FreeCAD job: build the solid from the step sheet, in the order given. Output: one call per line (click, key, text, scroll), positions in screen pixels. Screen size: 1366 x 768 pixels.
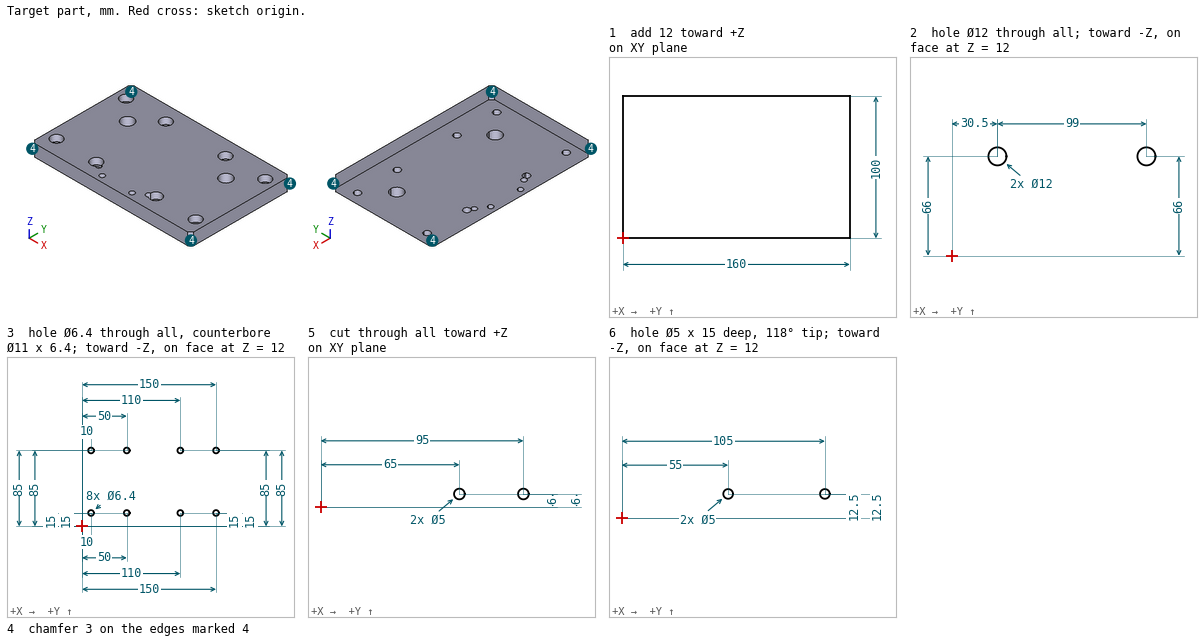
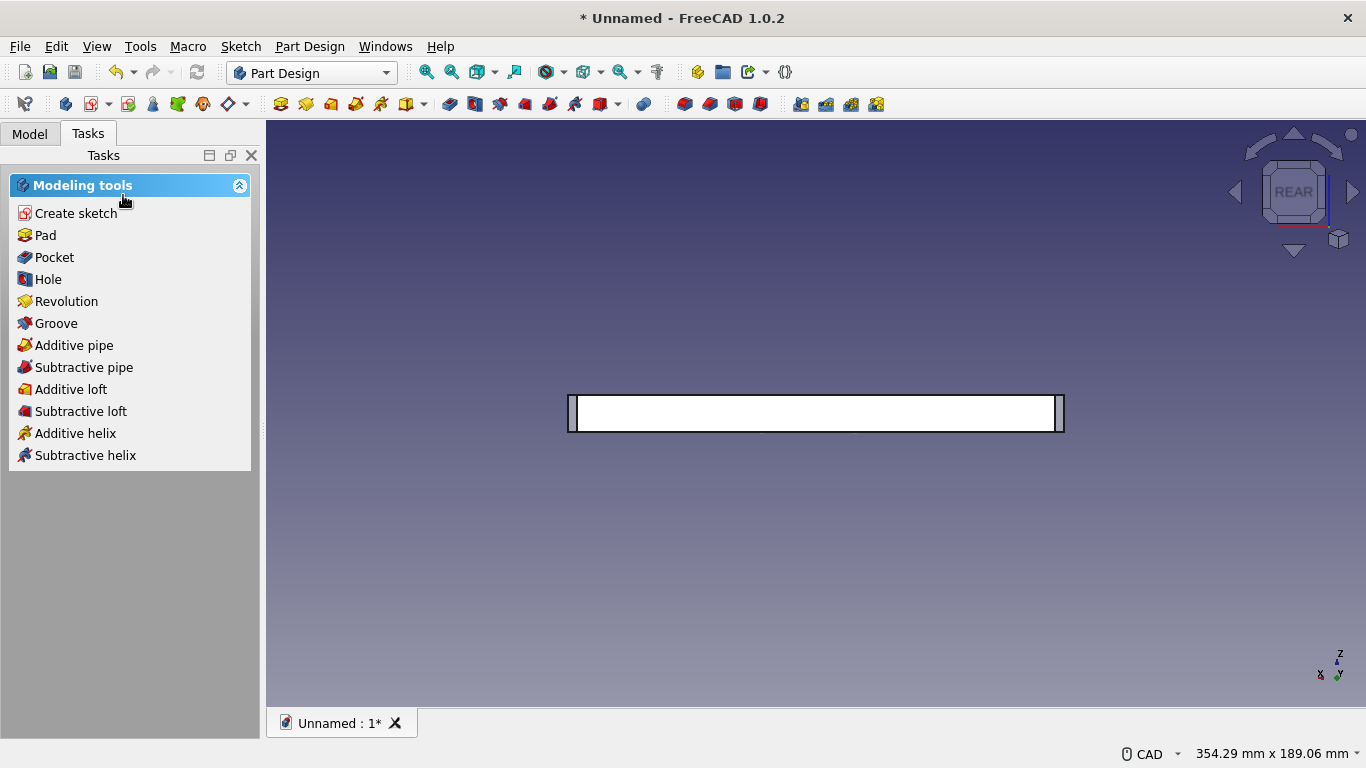
click(450, 104)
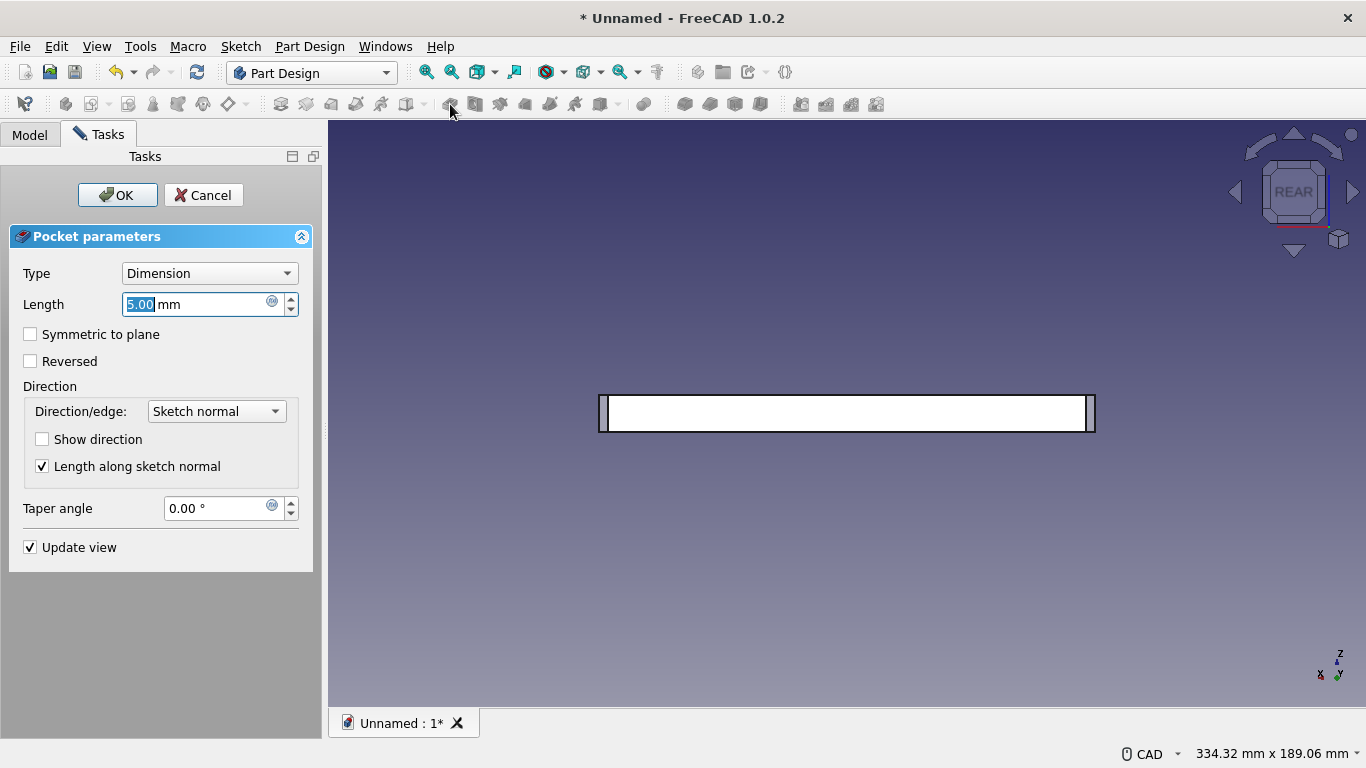
click(210, 274)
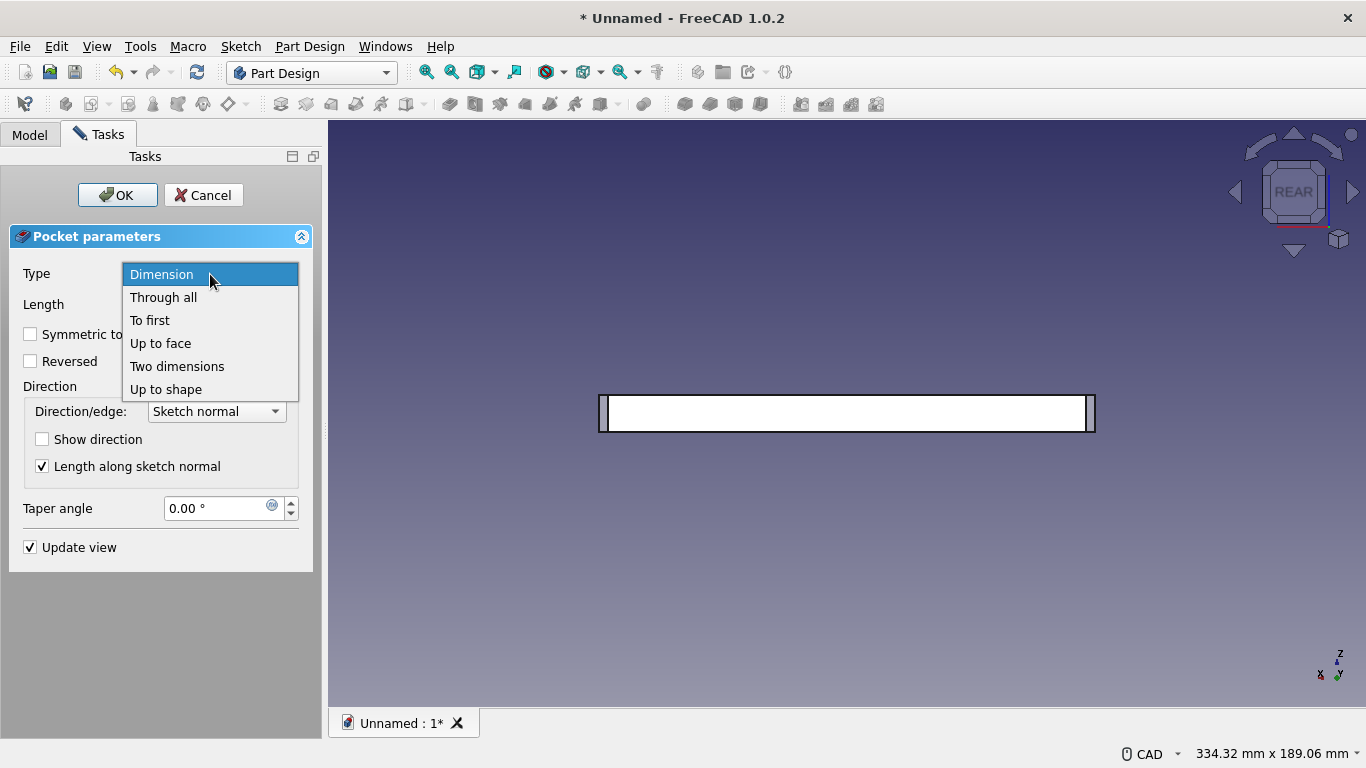
click(208, 298)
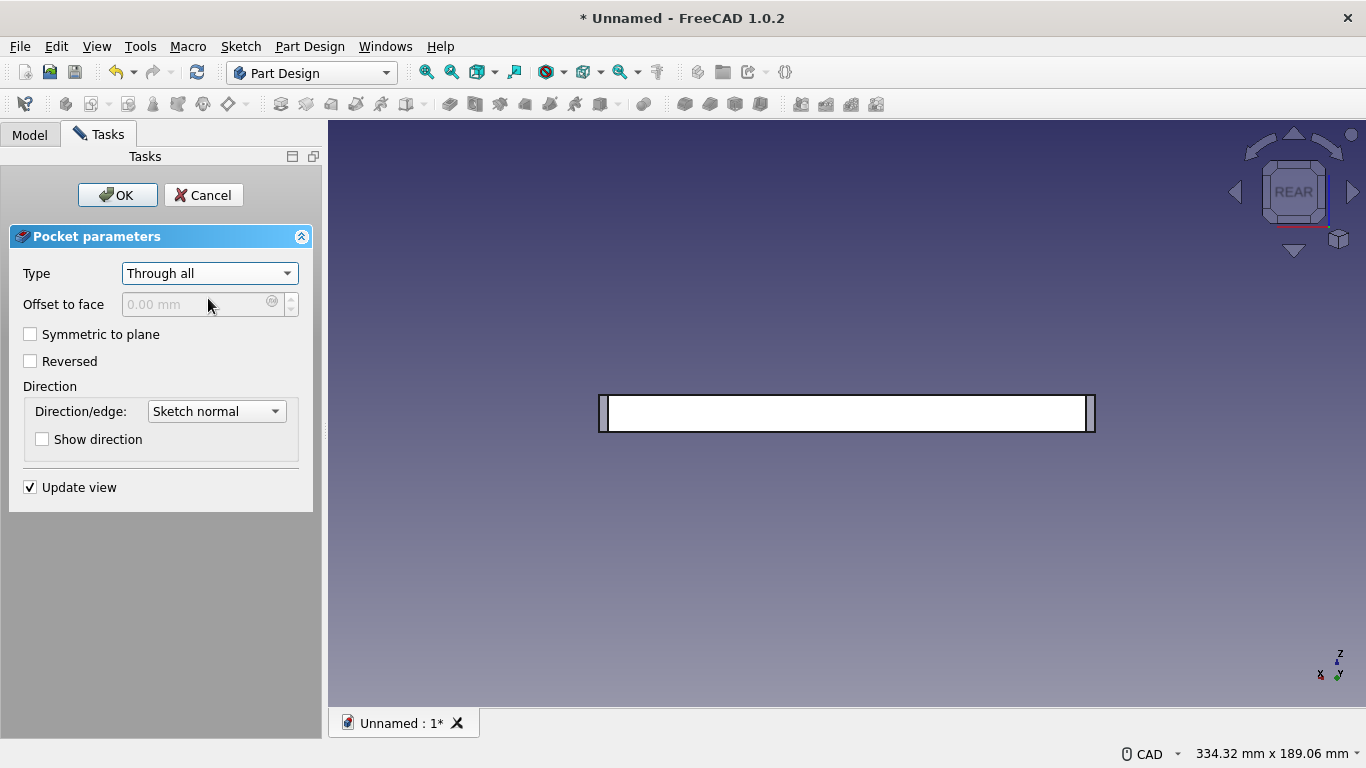
click(31, 361)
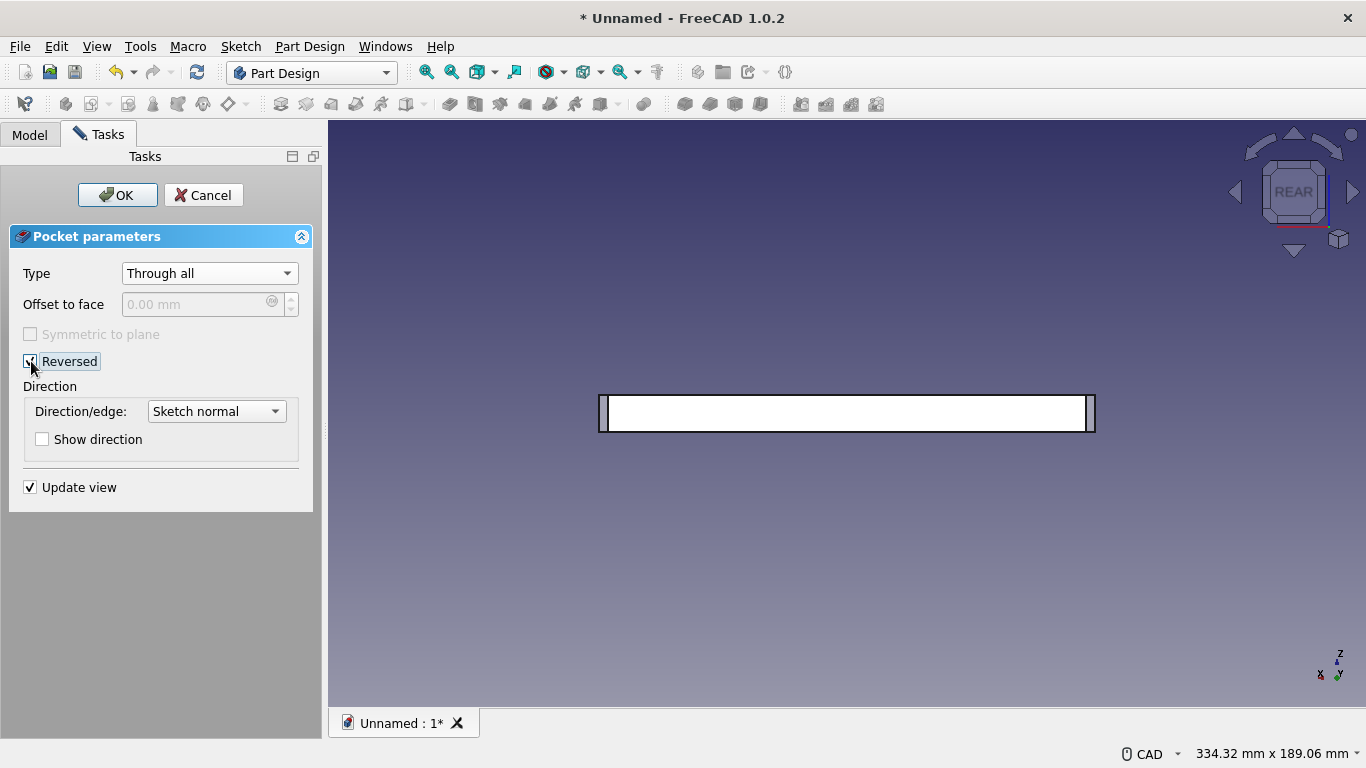
click(118, 195)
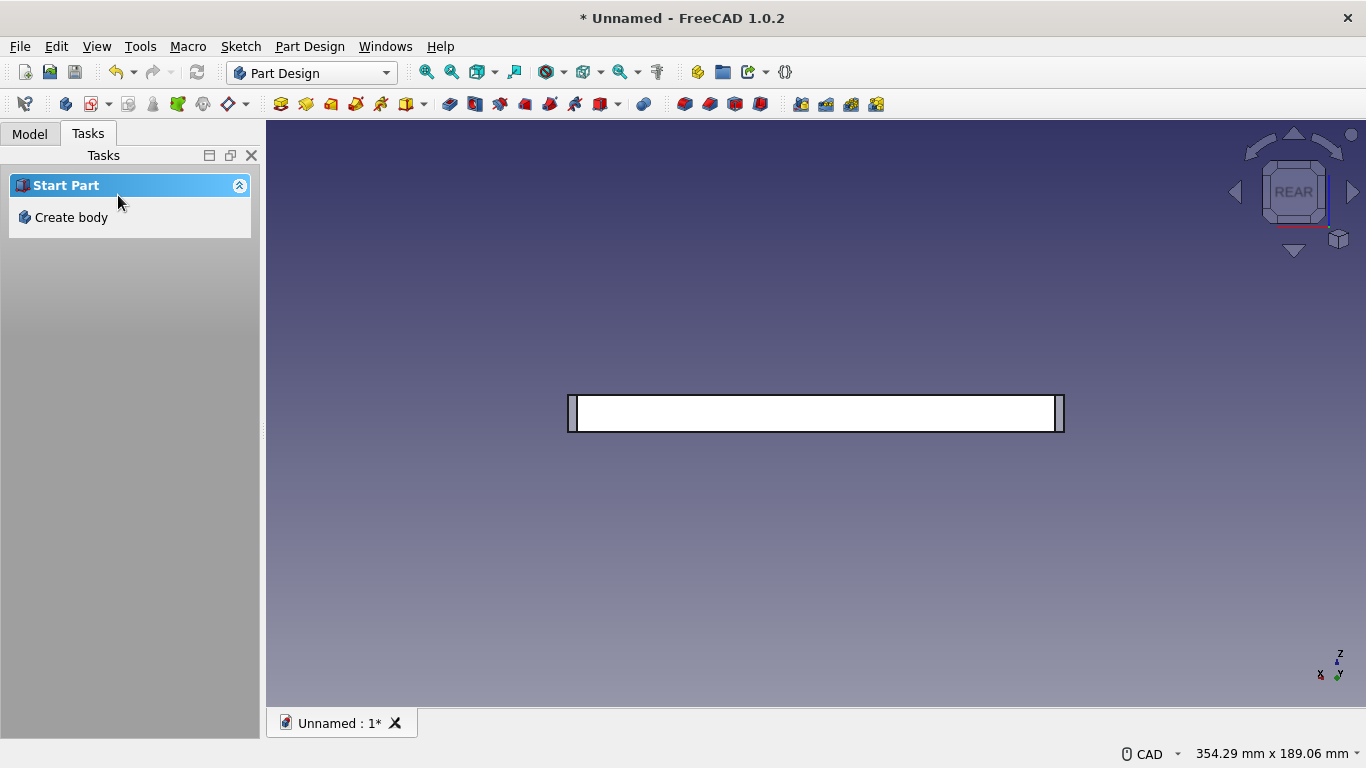
key(0)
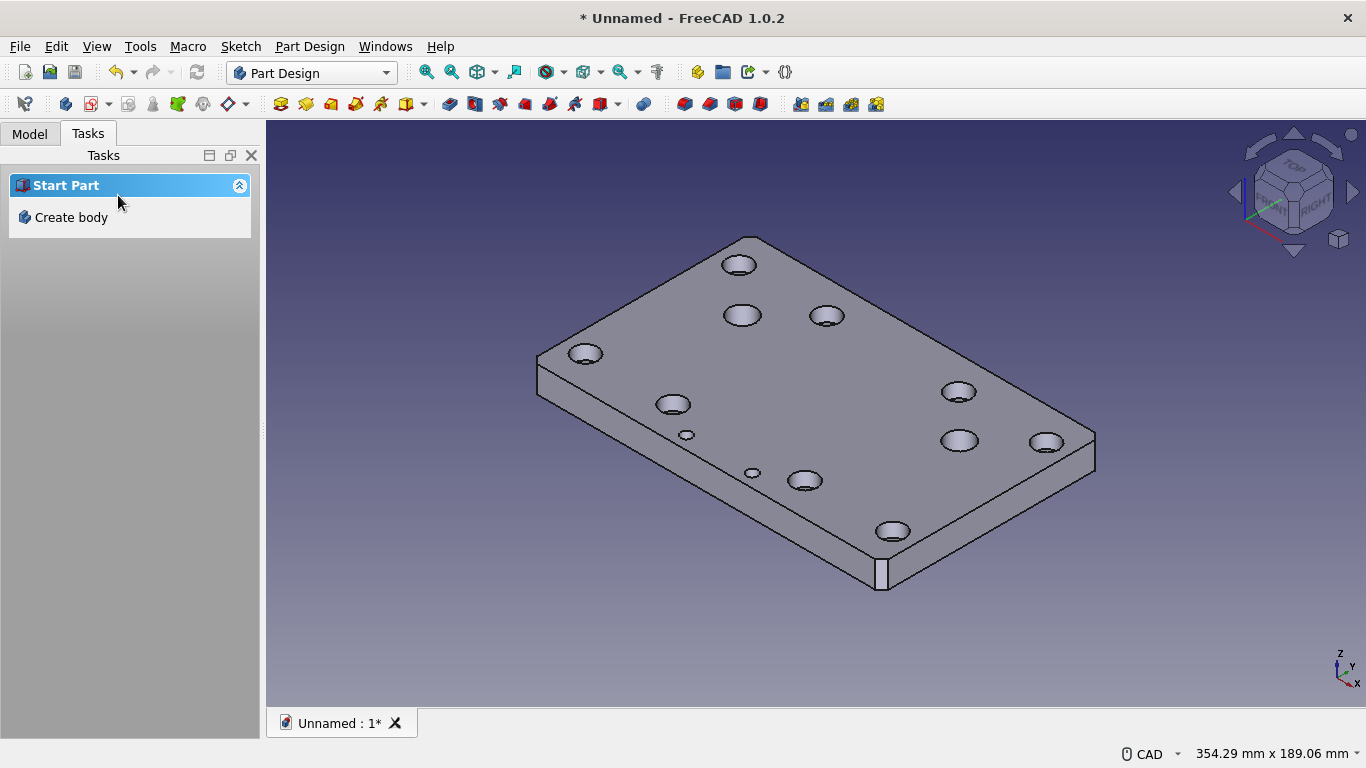
click(816, 397)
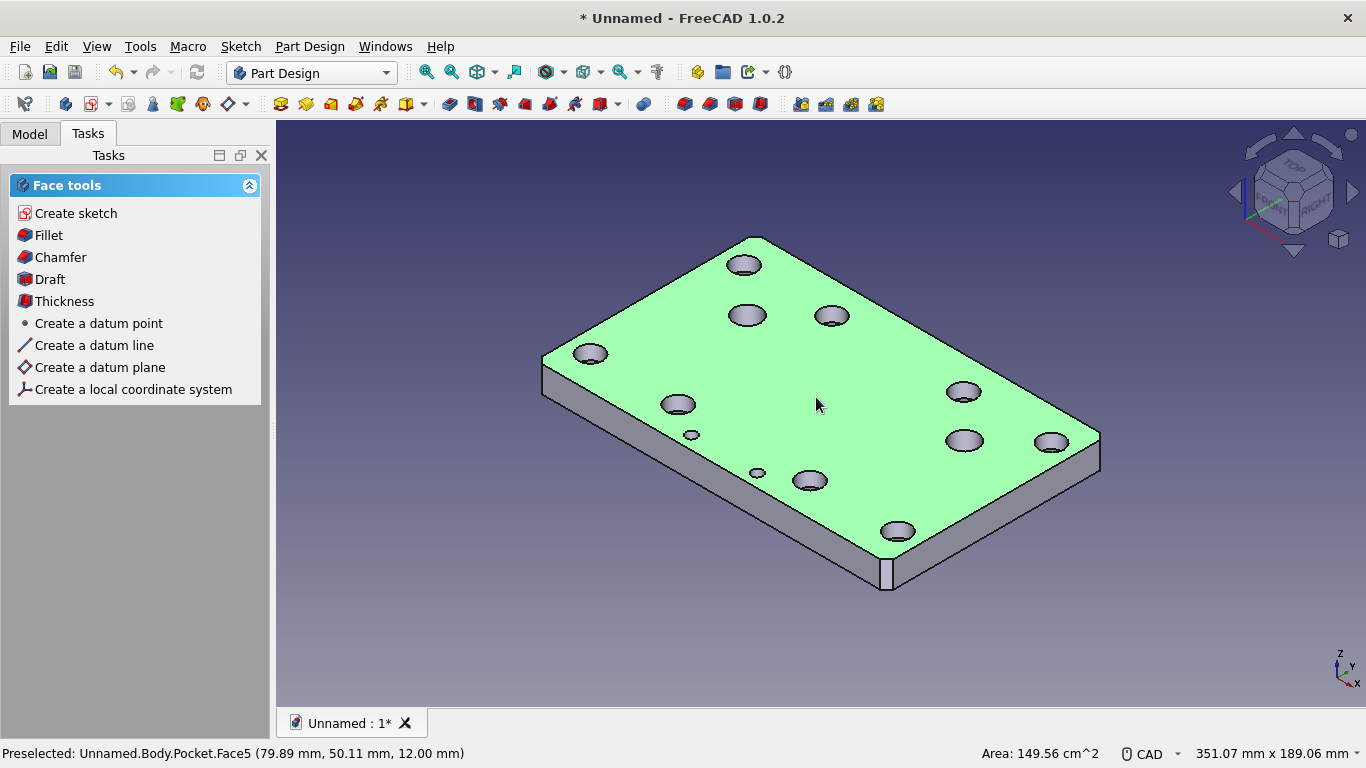
click(90, 104)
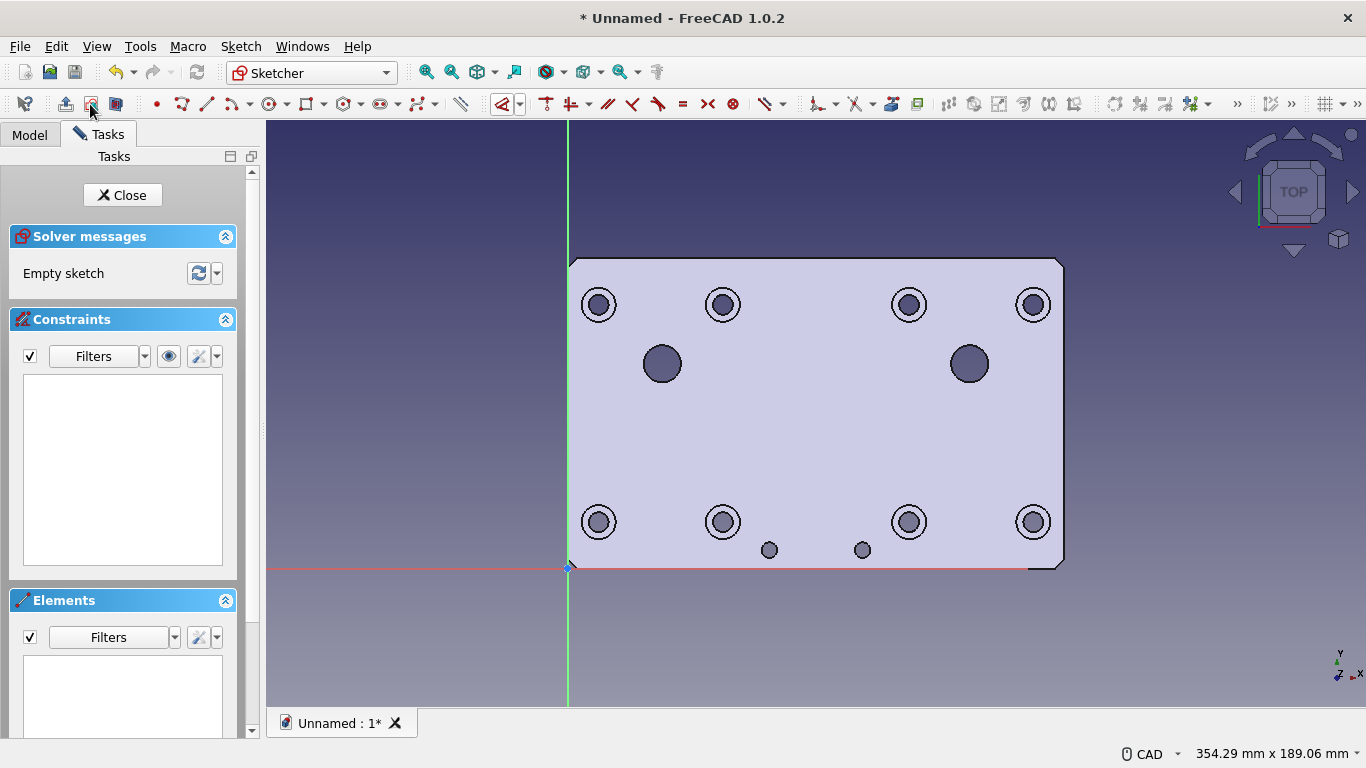
scroll(719, 679, up, 3)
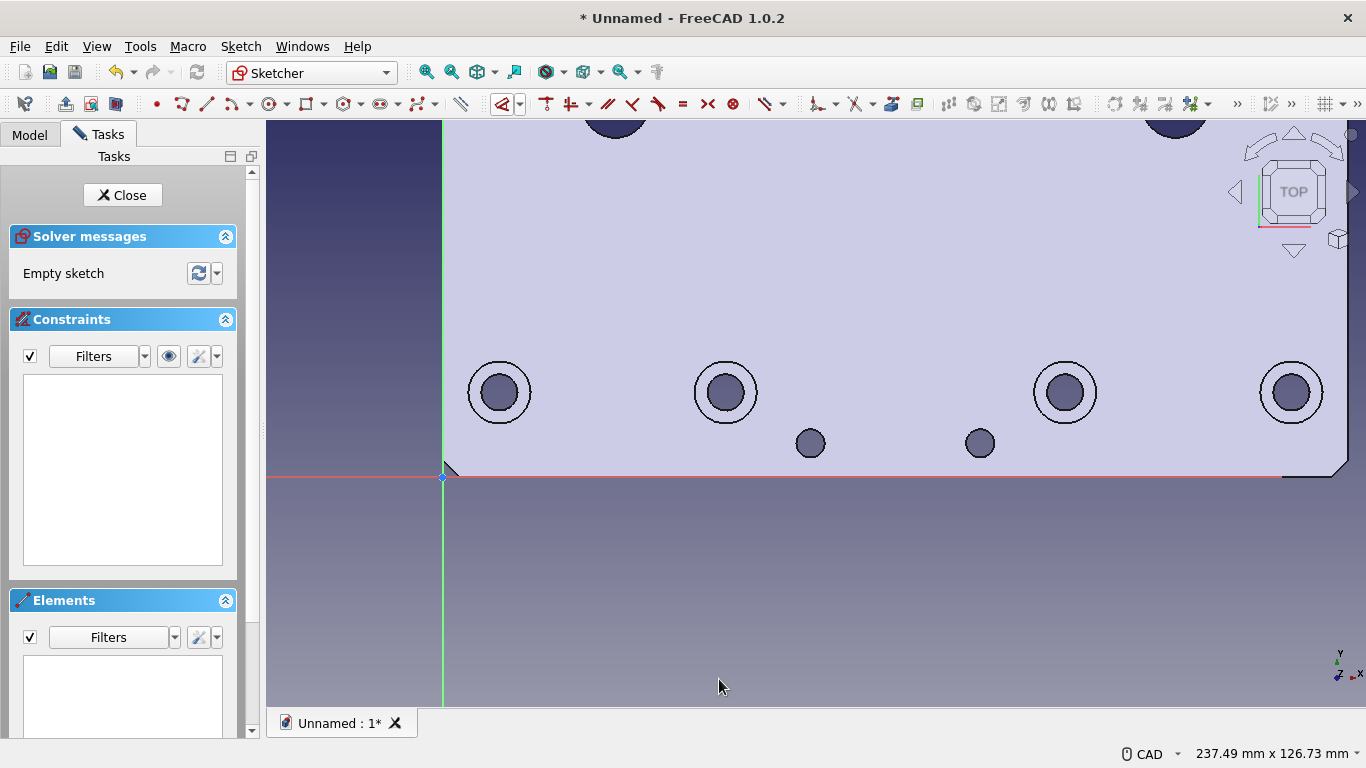
key(g)
key(c)